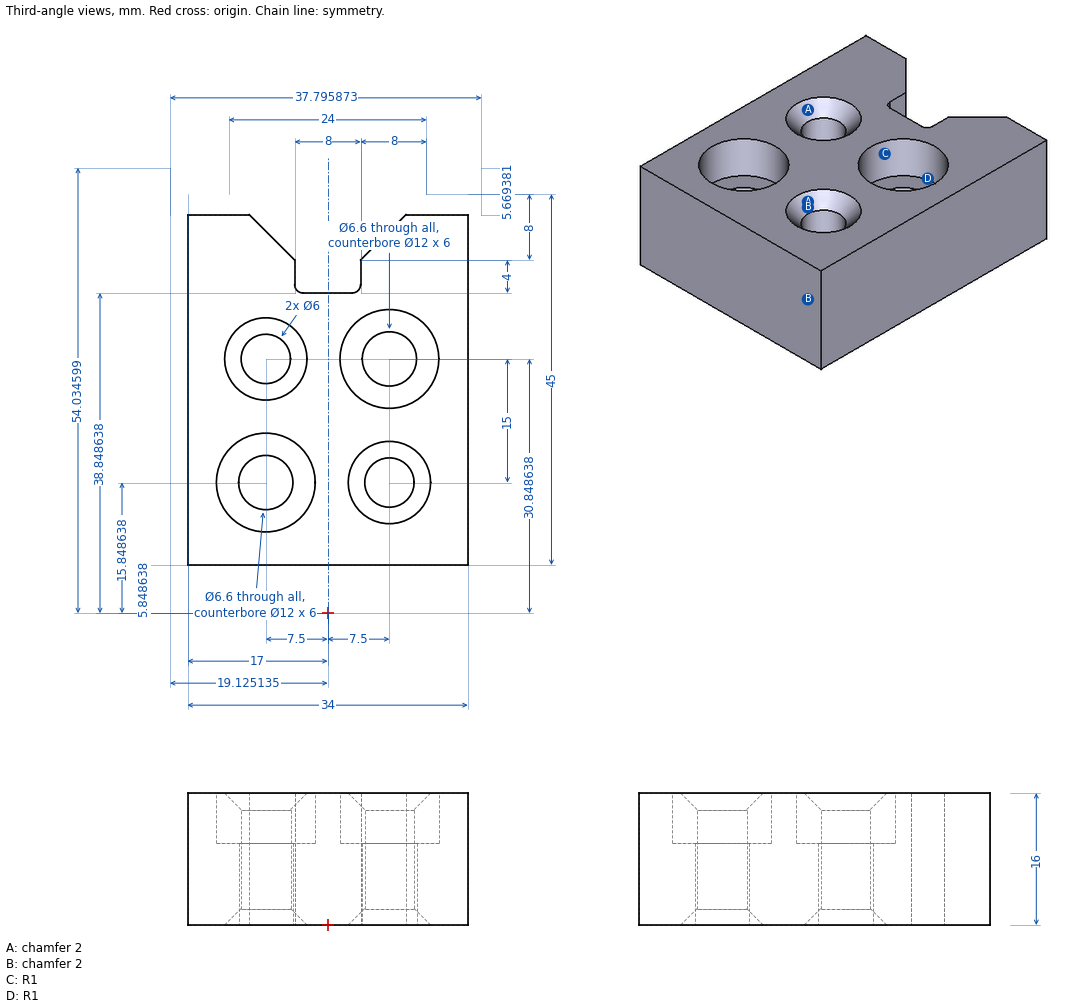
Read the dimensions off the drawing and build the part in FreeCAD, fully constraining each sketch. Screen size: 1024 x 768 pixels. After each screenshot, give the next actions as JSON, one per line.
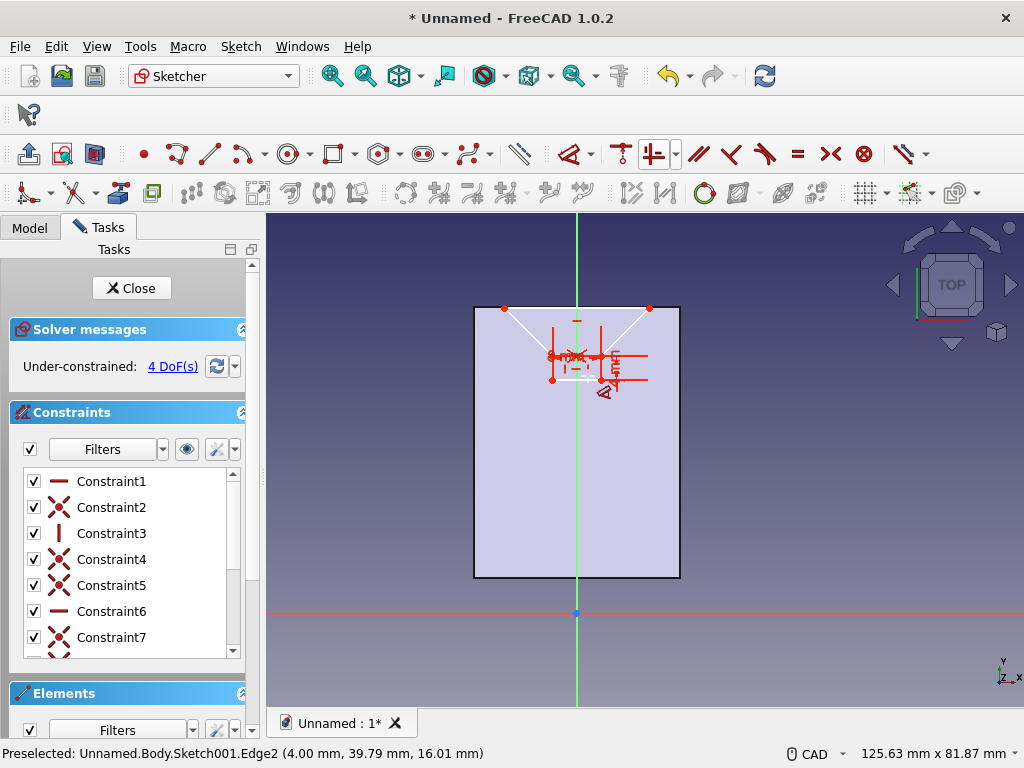
{"action": "left_click", "coordinate": [606, 308]}
{"action": "left_click", "coordinate": [544, 274]}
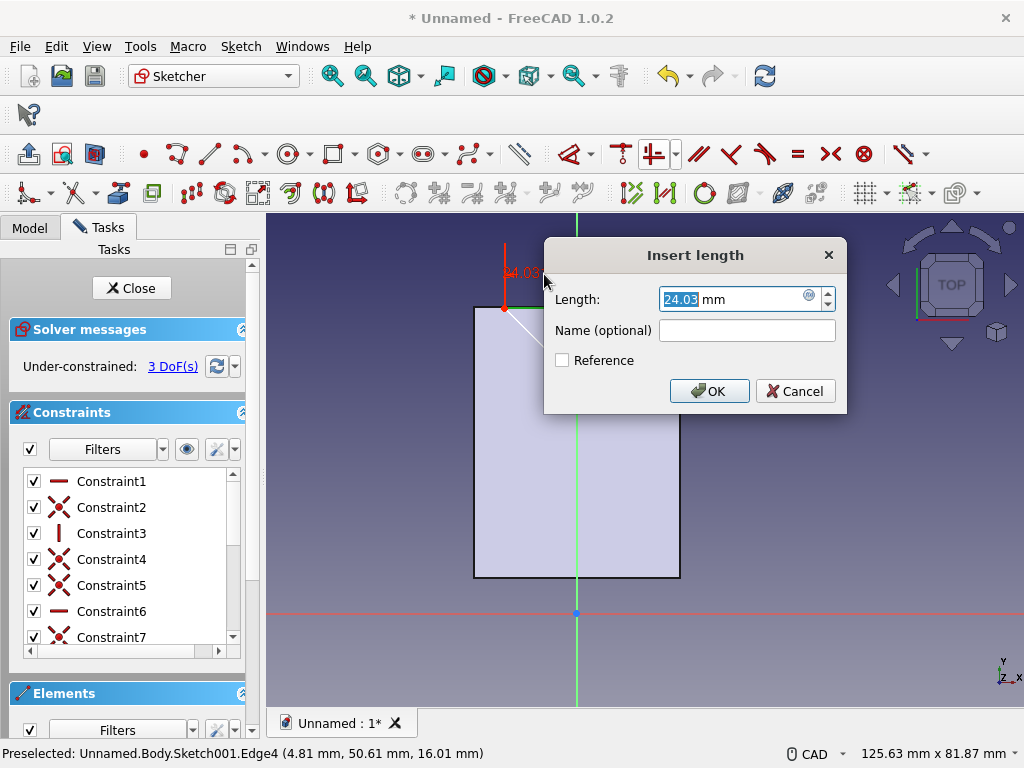
{"action": "type", "text": "24"}
{"action": "key", "text": "Return"}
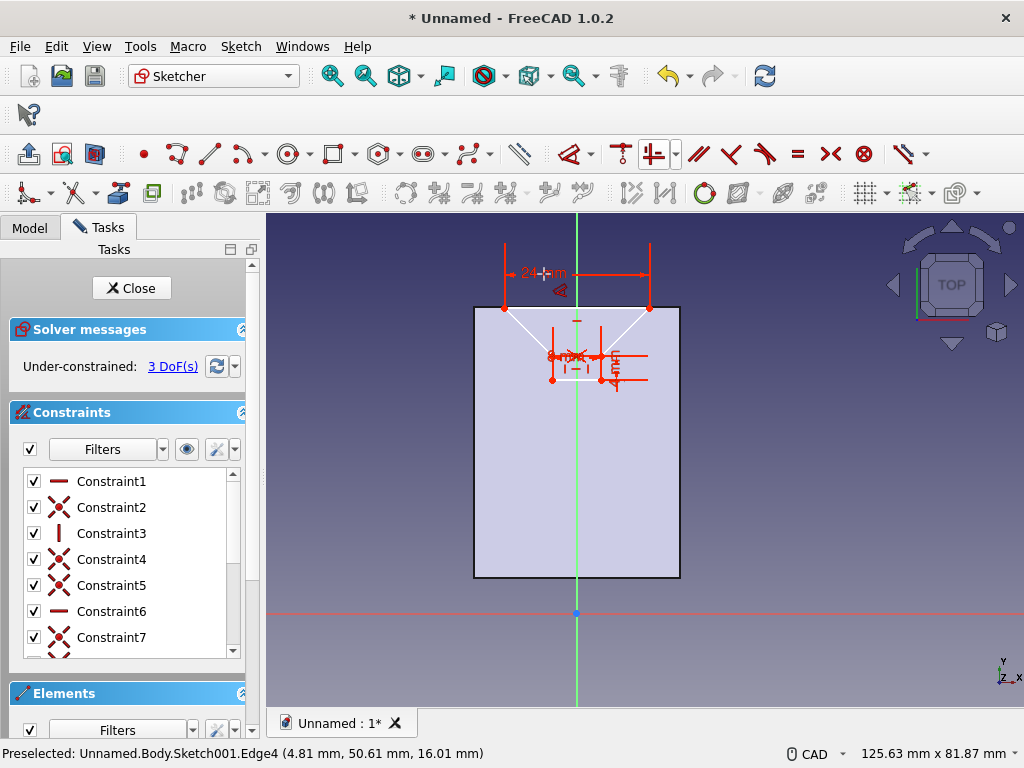
{"action": "left_click", "coordinate": [616, 342]}
{"action": "left_click", "coordinate": [625, 274]}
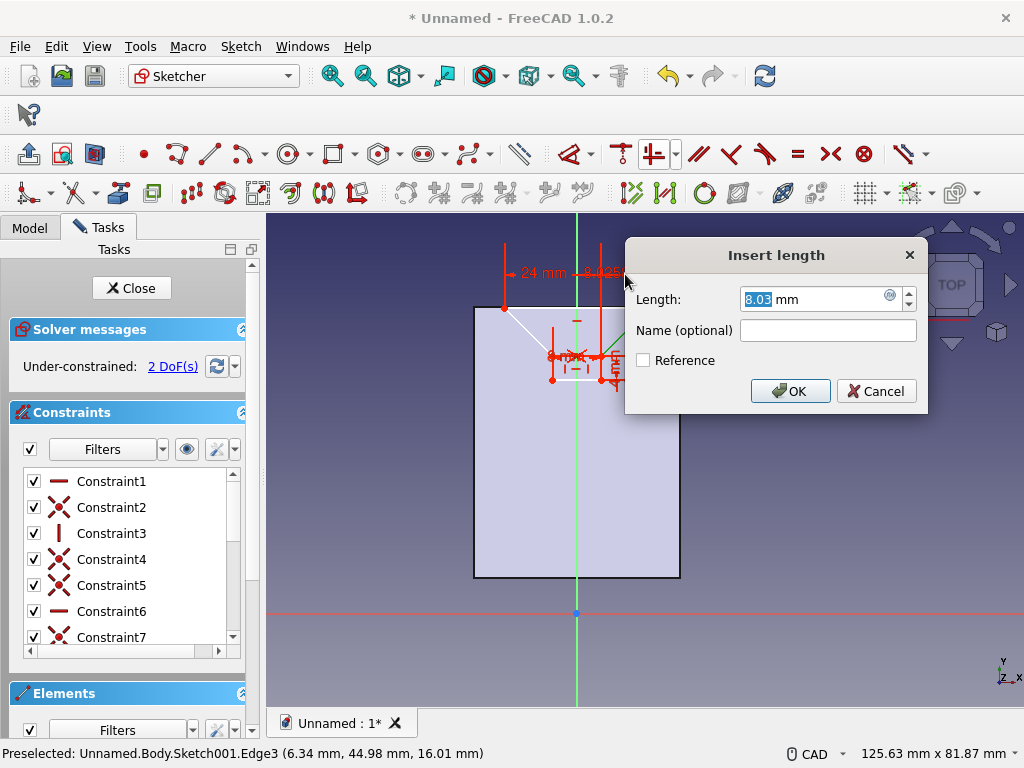
{"action": "type", "text": "8"}
{"action": "key", "text": "Return"}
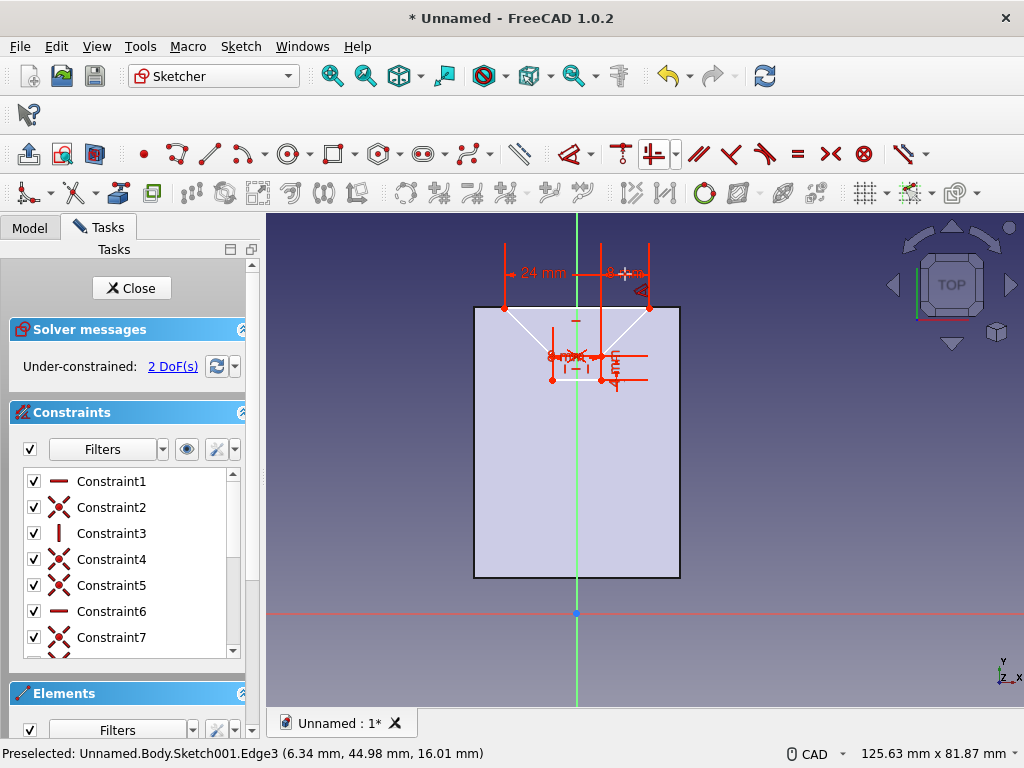
{"action": "left_click", "coordinate": [616, 342]}
{"action": "left_click", "coordinate": [683, 332]}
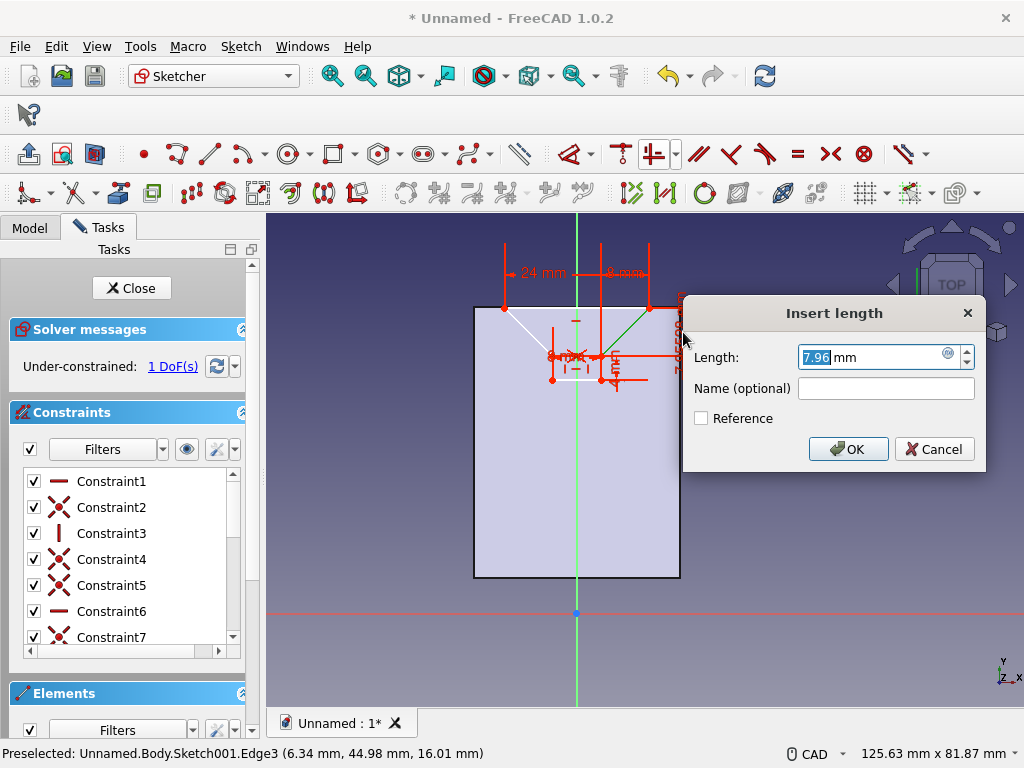
{"action": "type", "text": "8"}
{"action": "key", "text": "Return"}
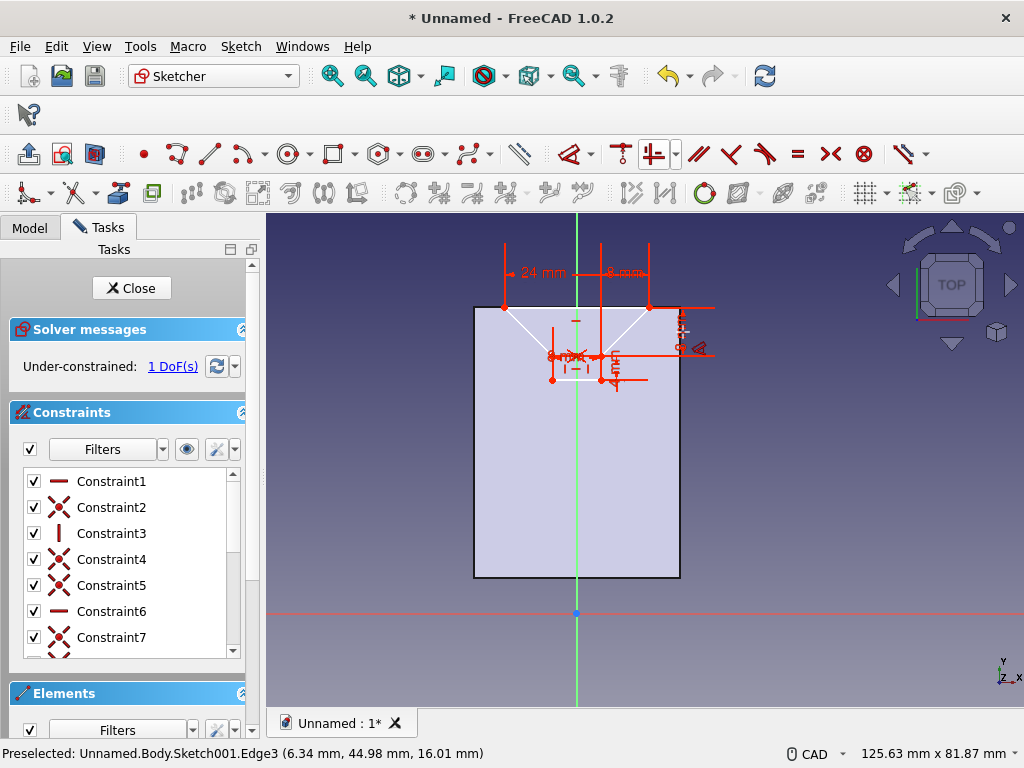
{"action": "left_click", "coordinate": [553, 380]}
{"action": "left_click", "coordinate": [519, 497]}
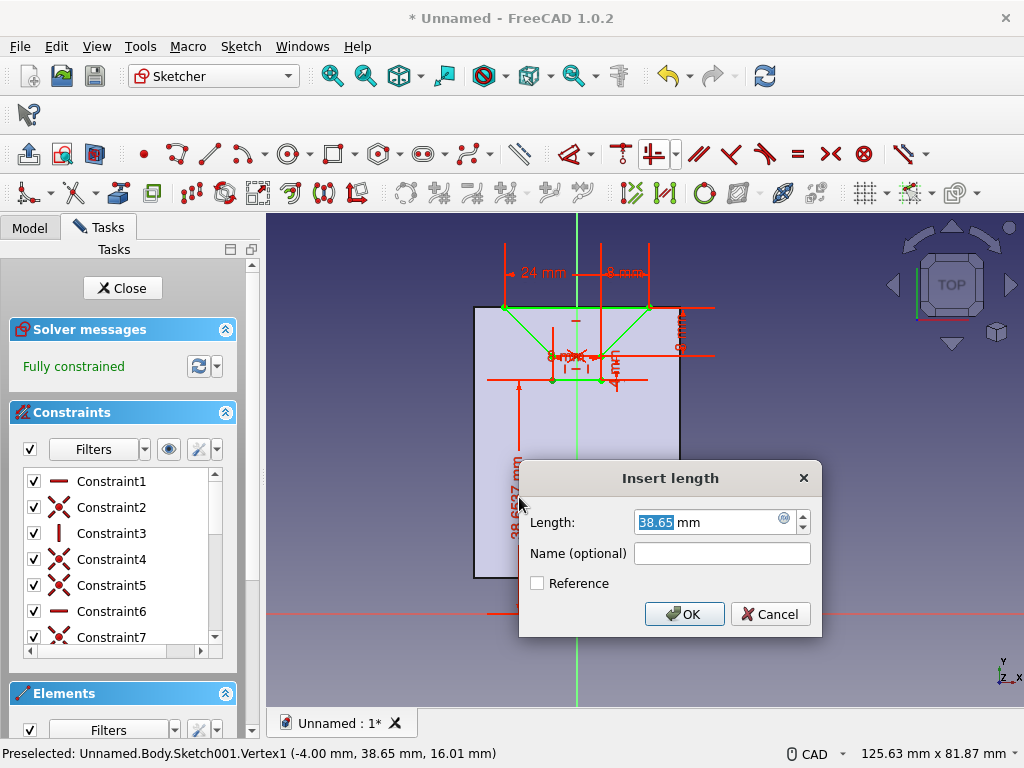
{"action": "type", "text": "38.848638"}
{"action": "key", "text": "Return"}
{"action": "key", "text": "Escape"}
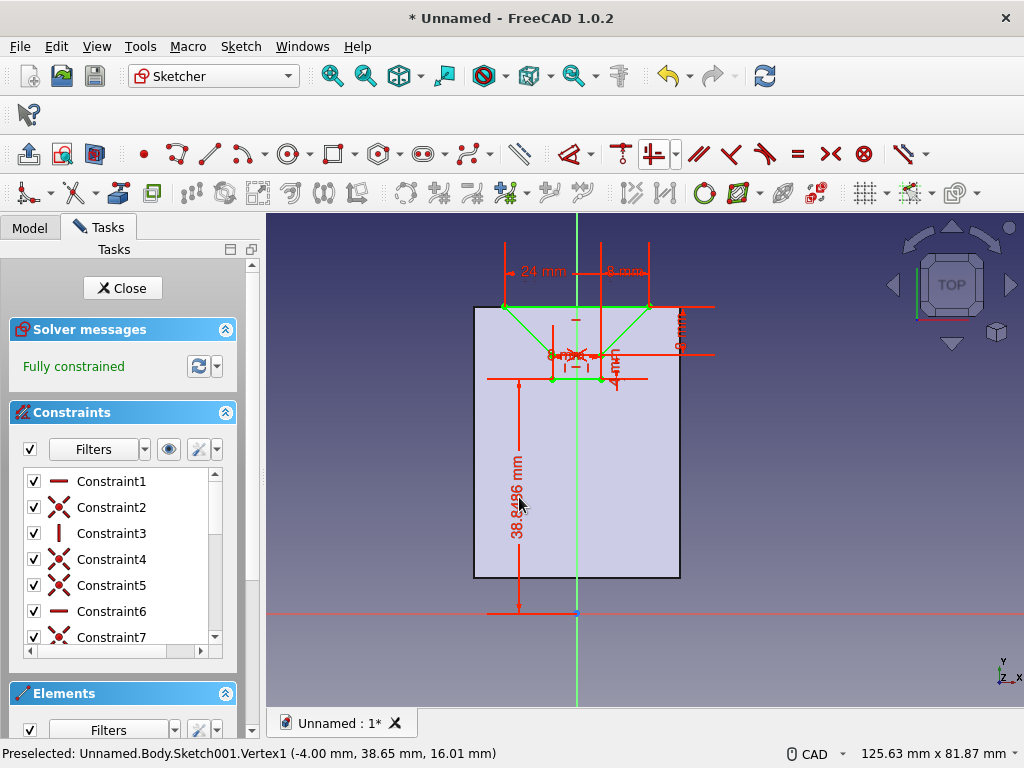
{"action": "left_click", "coordinate": [123, 288]}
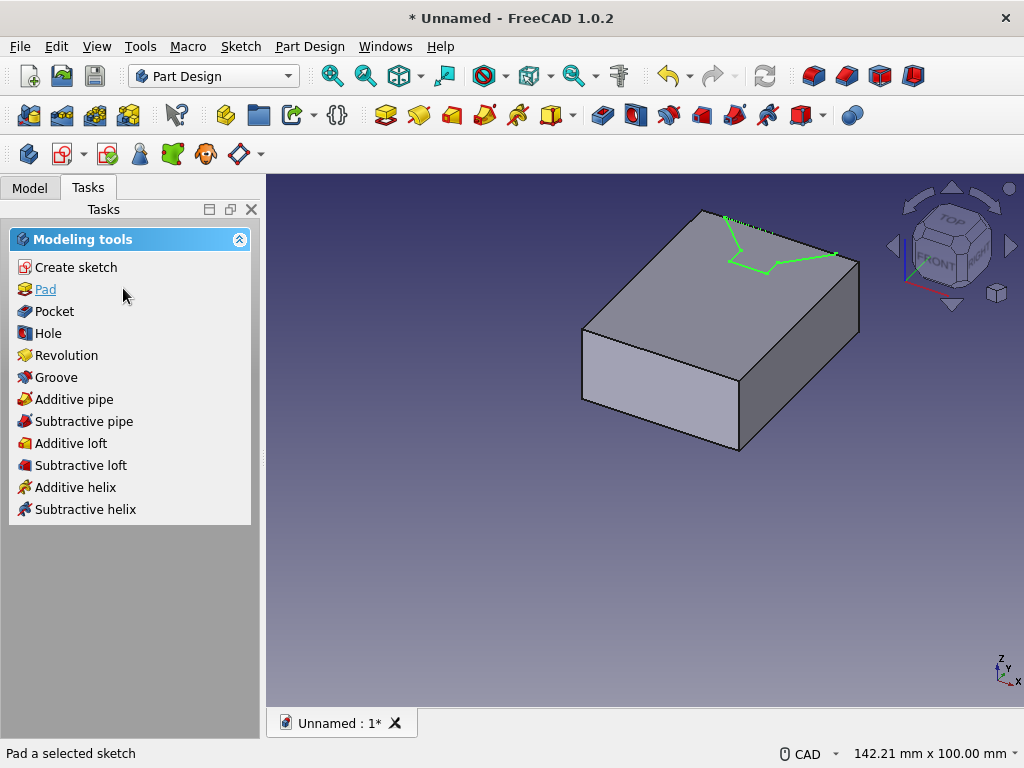
{"action": "left_click", "coordinate": [603, 116]}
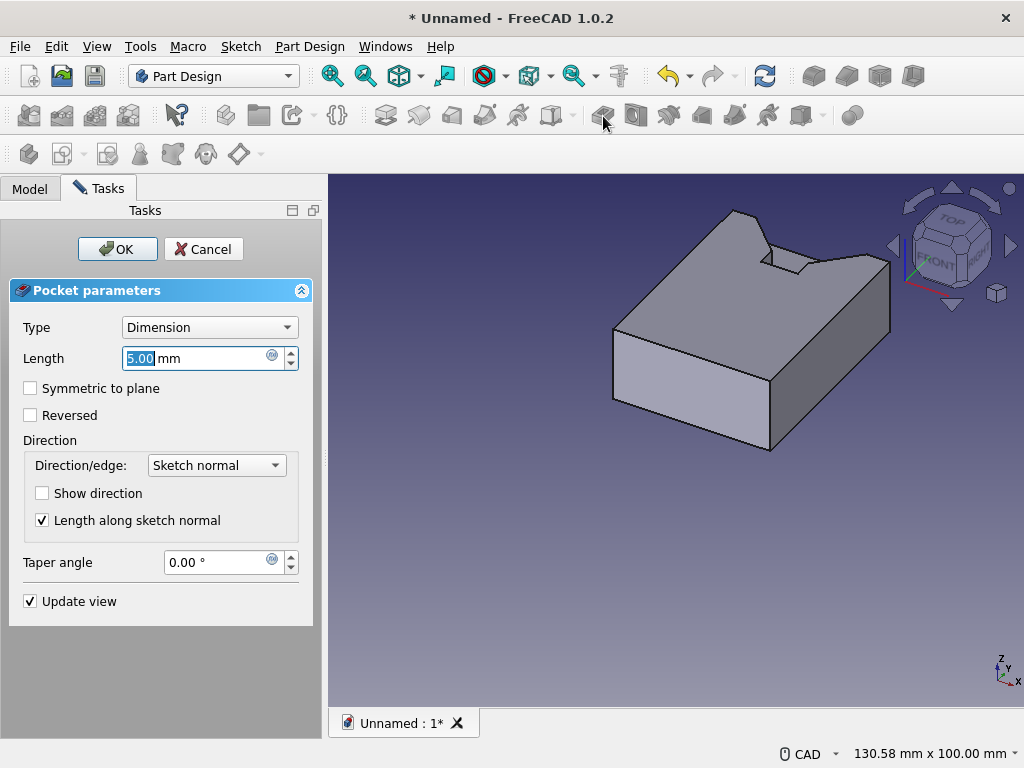
{"action": "left_click", "coordinate": [210, 328]}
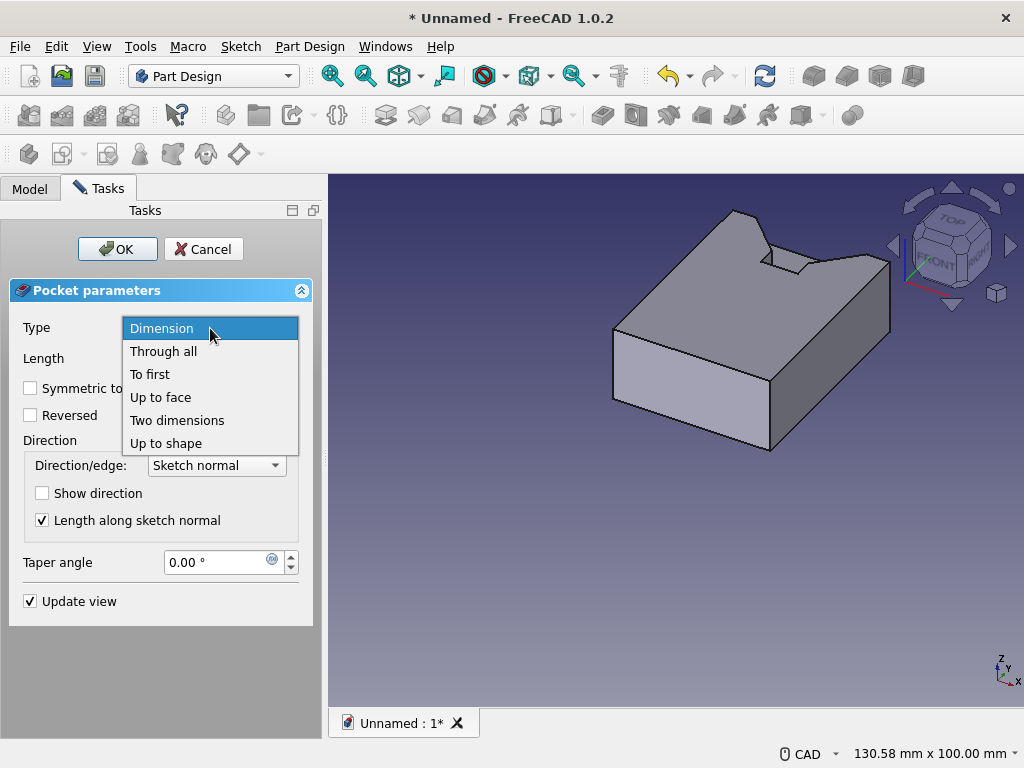
{"action": "left_click", "coordinate": [208, 352]}